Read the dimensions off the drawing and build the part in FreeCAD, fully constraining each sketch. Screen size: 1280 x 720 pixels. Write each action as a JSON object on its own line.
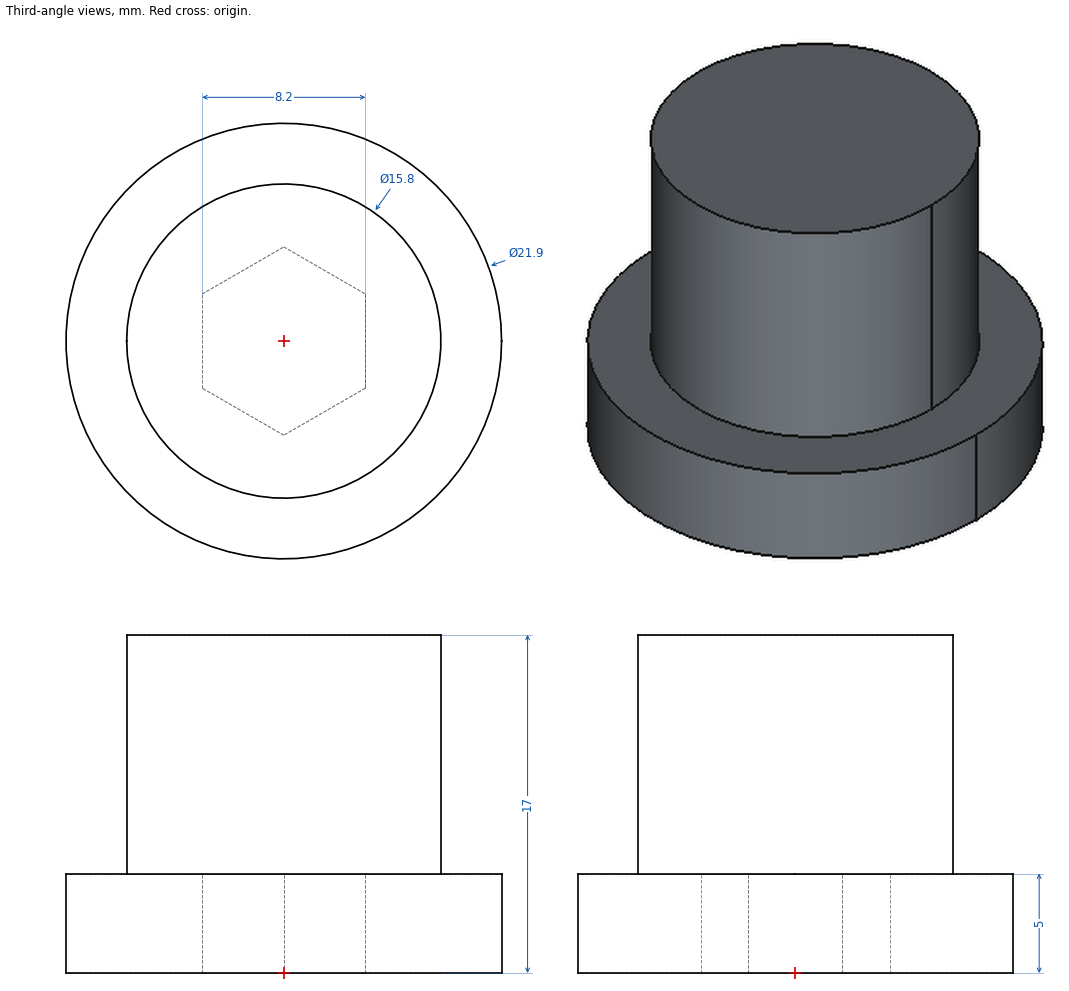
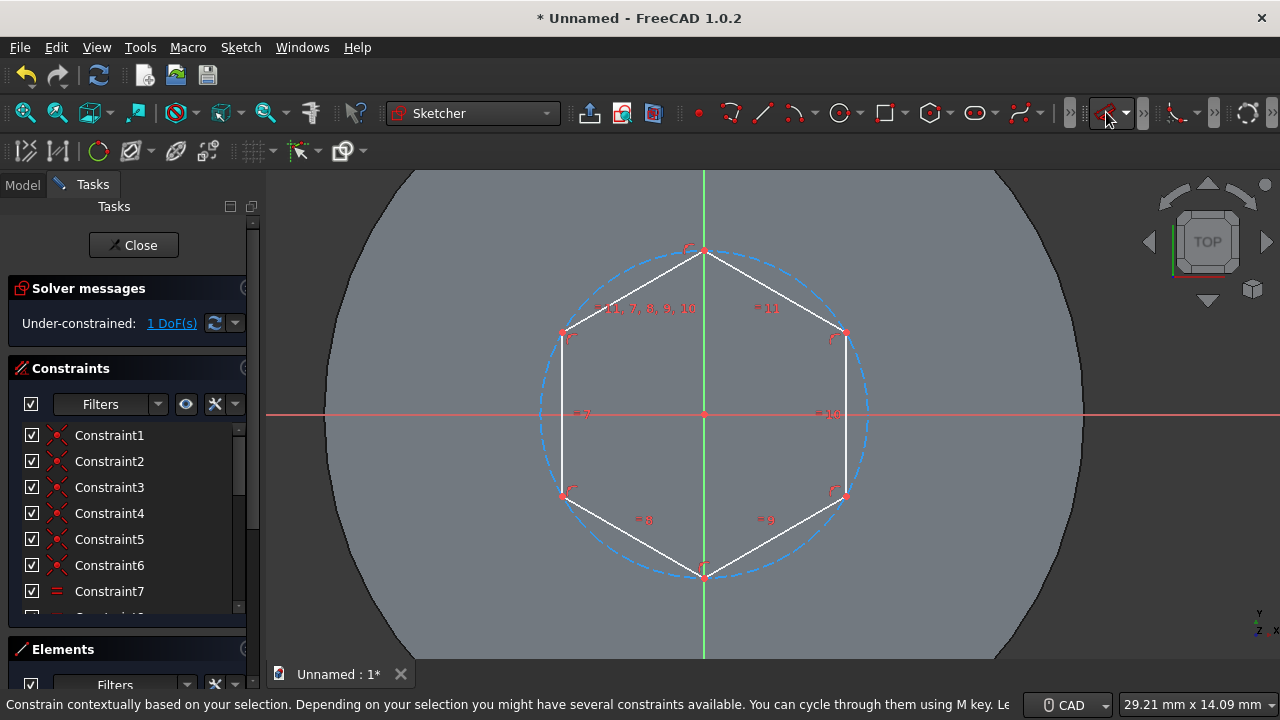
{"action": "left_click", "coordinate": [562, 333]}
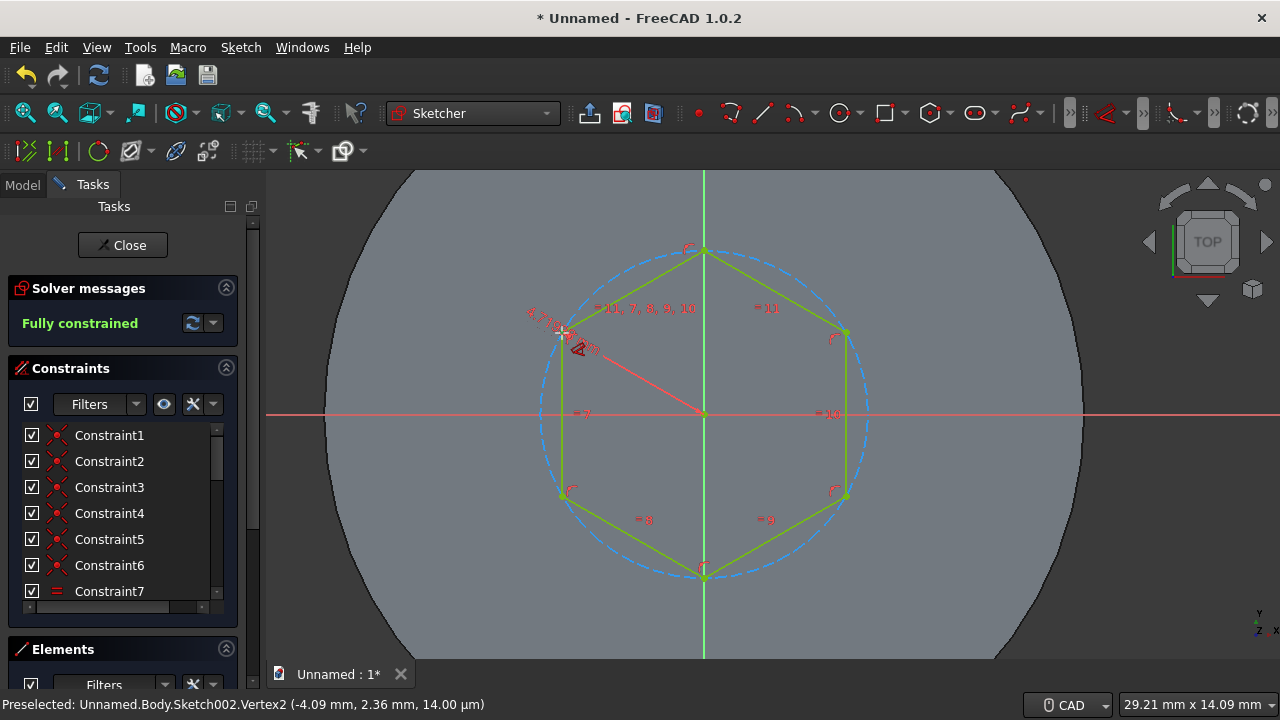
{"action": "left_click", "coordinate": [846, 496]}
{"action": "left_click", "coordinate": [605, 578]}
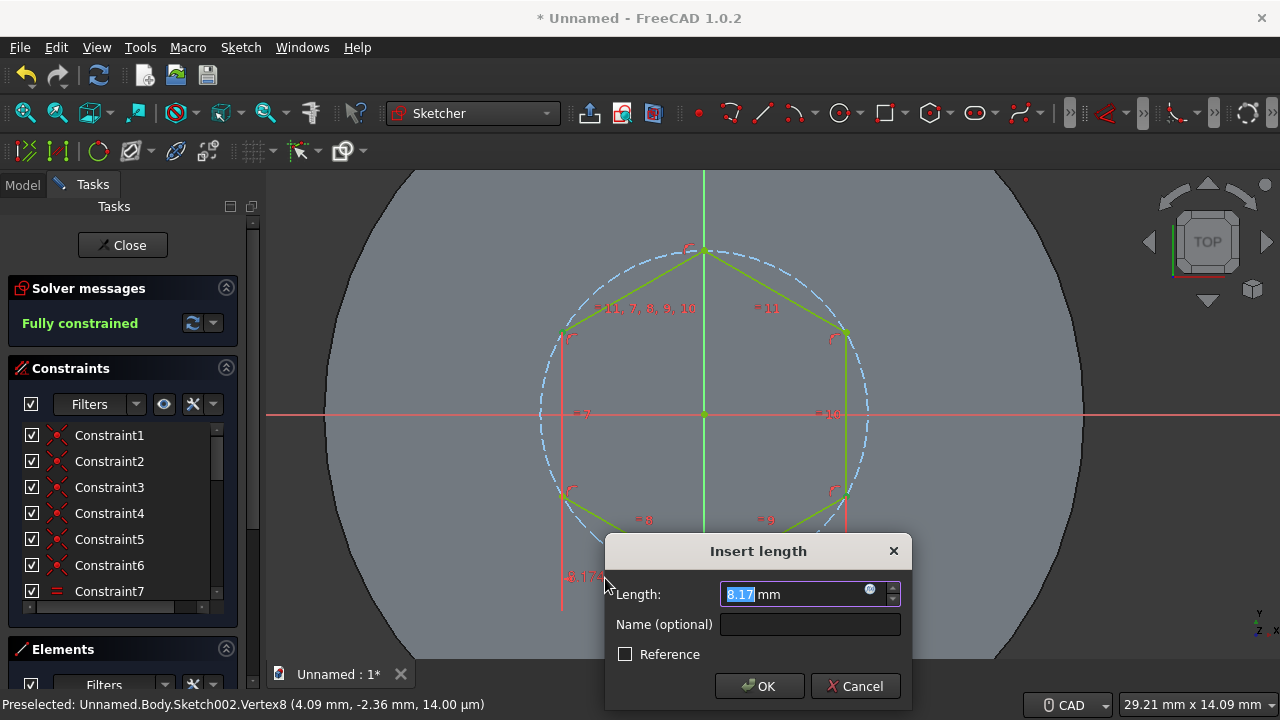
{"action": "type", "text": "8.2"}
{"action": "key", "text": "Return"}
{"action": "key", "text": "Escape"}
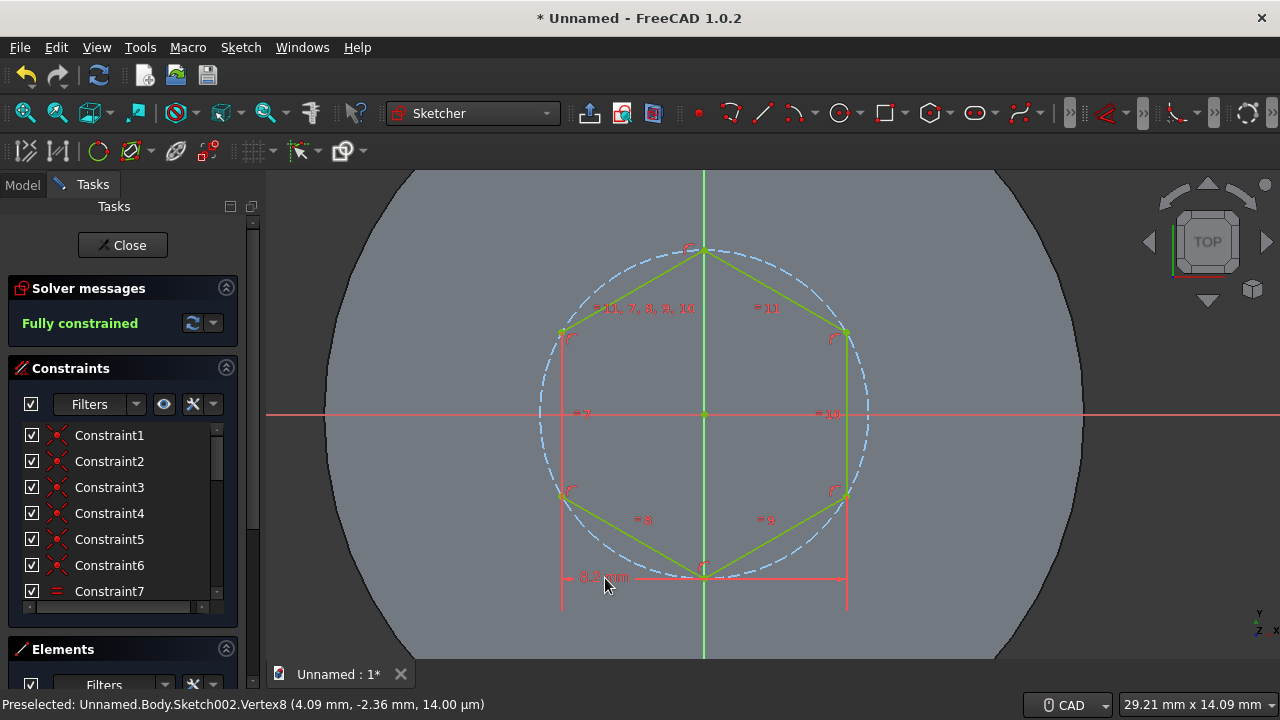
{"action": "left_click", "coordinate": [123, 245]}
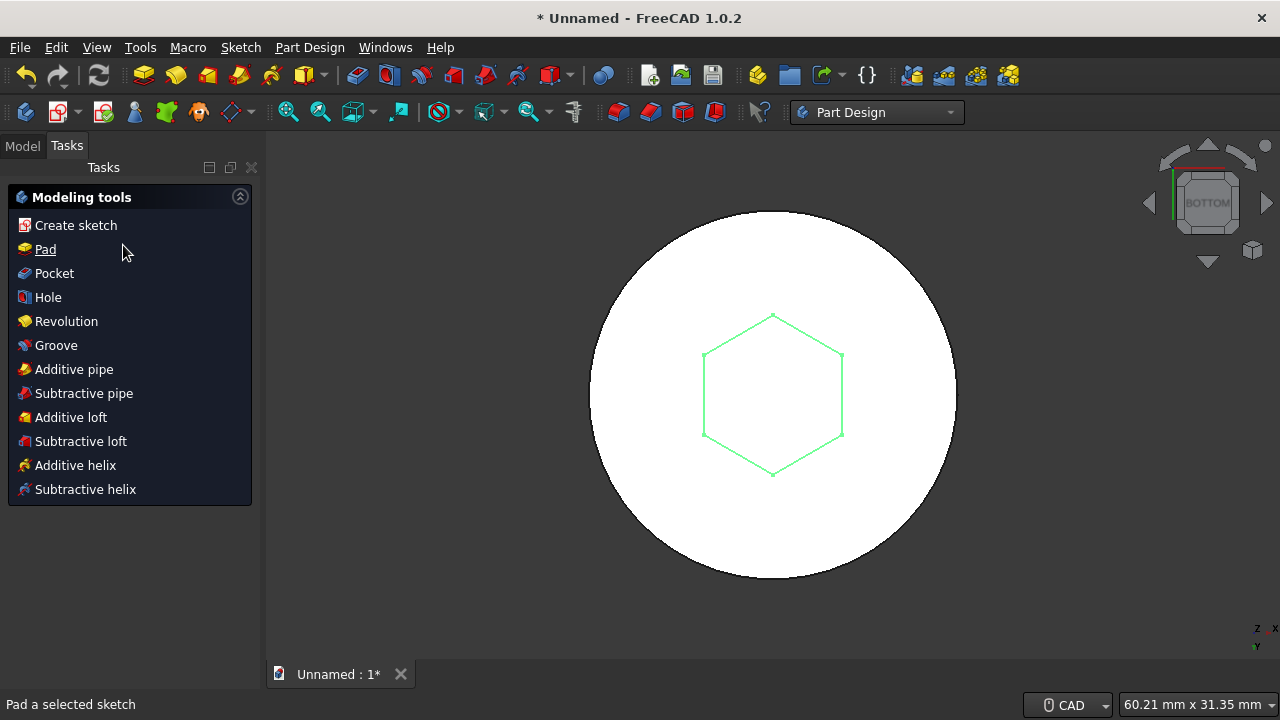
{"action": "left_click", "coordinate": [358, 76]}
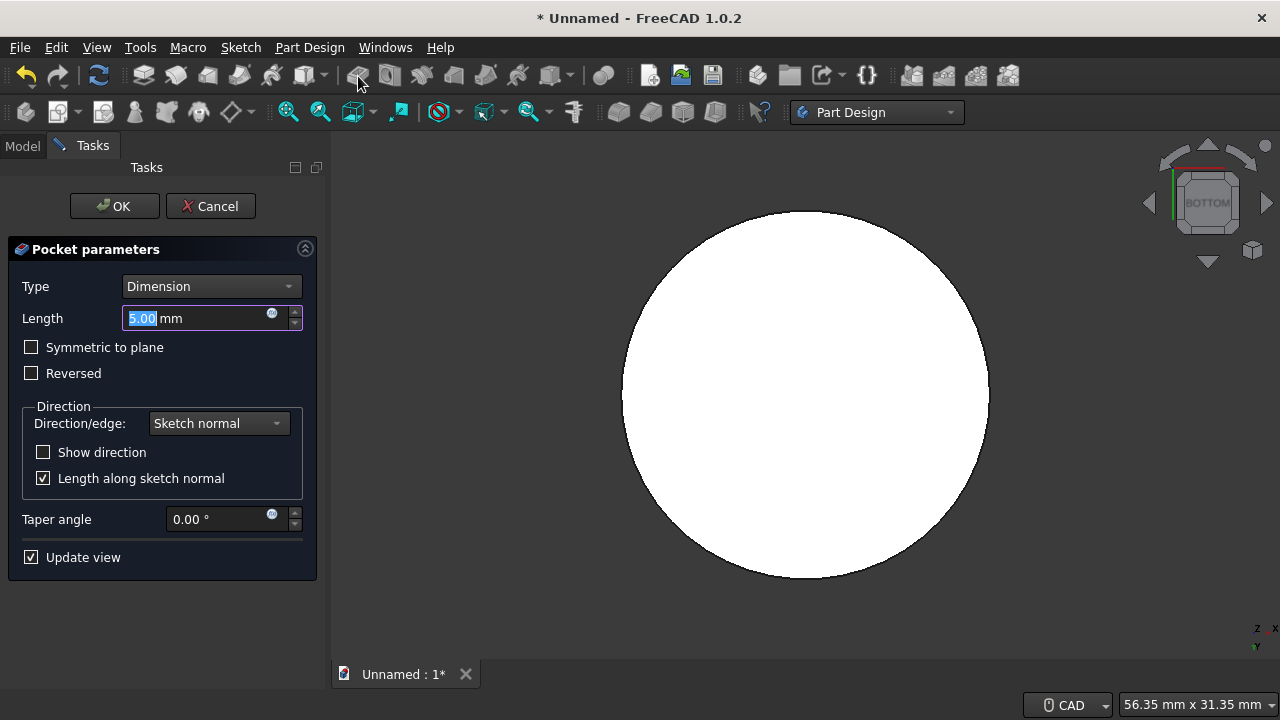
{"action": "type", "text": "5"}
{"action": "key", "text": "Tab"}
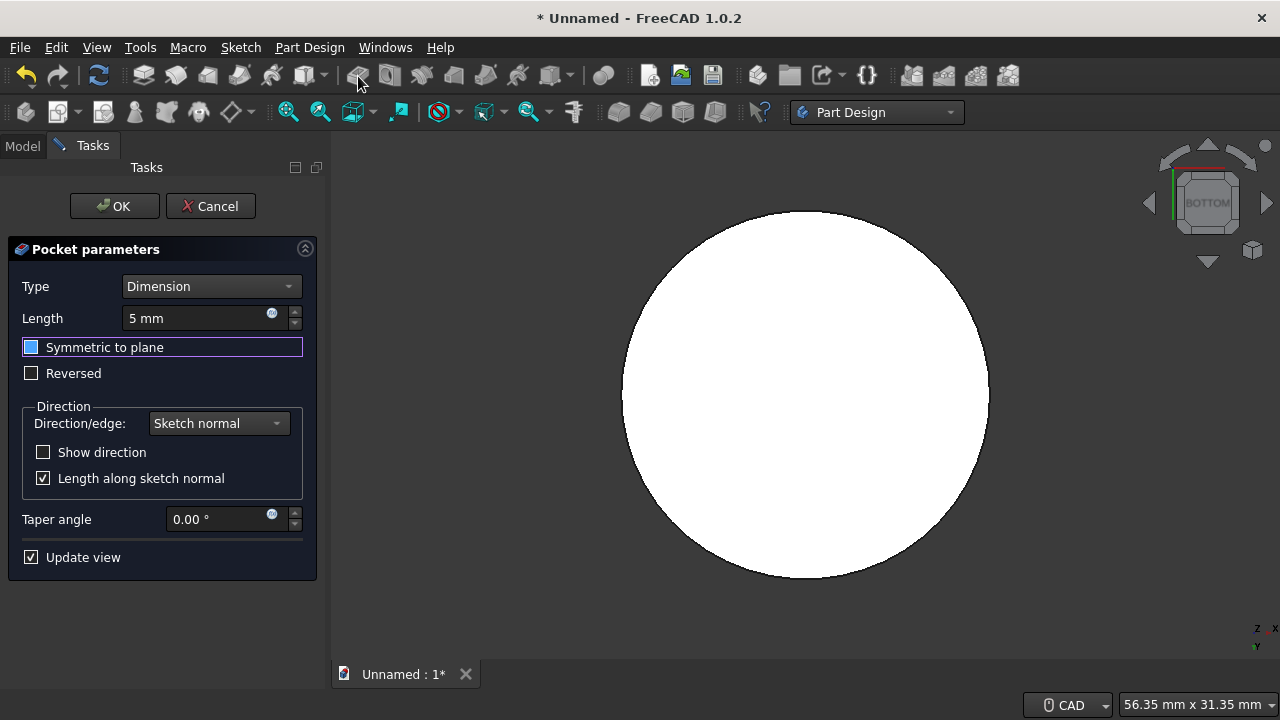
{"action": "left_click", "coordinate": [30, 373]}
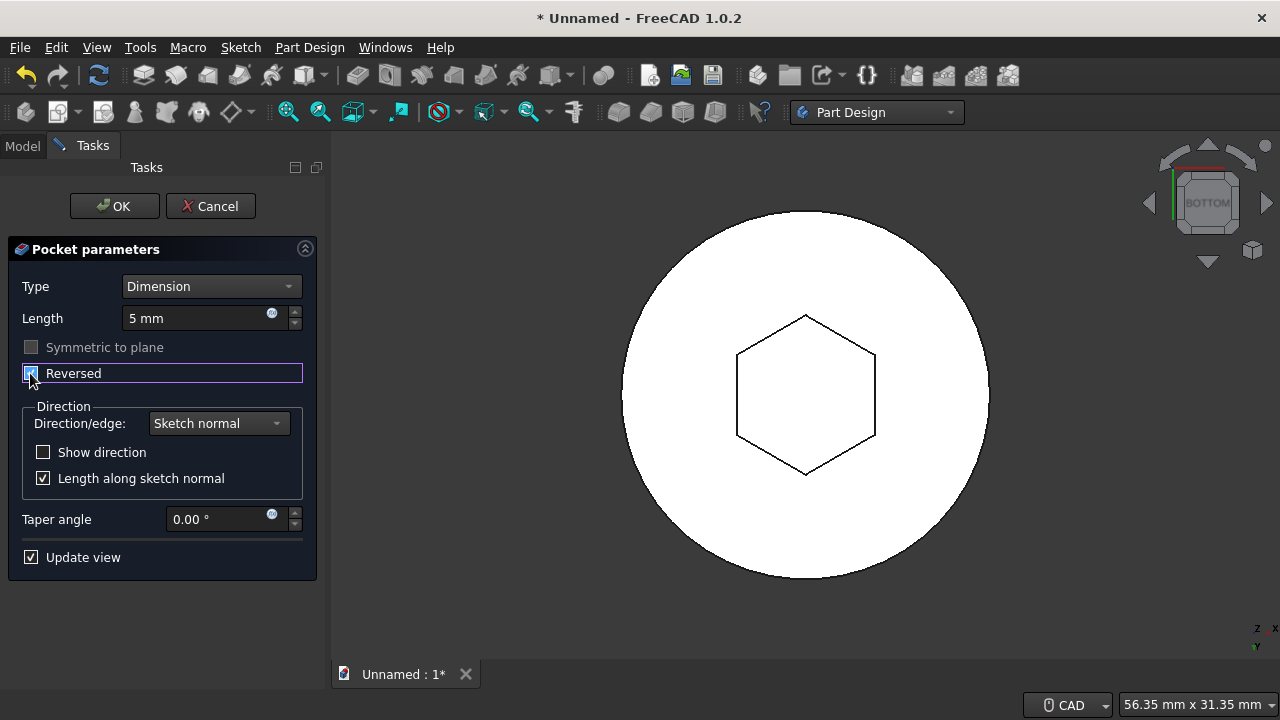
{"action": "left_click", "coordinate": [115, 206]}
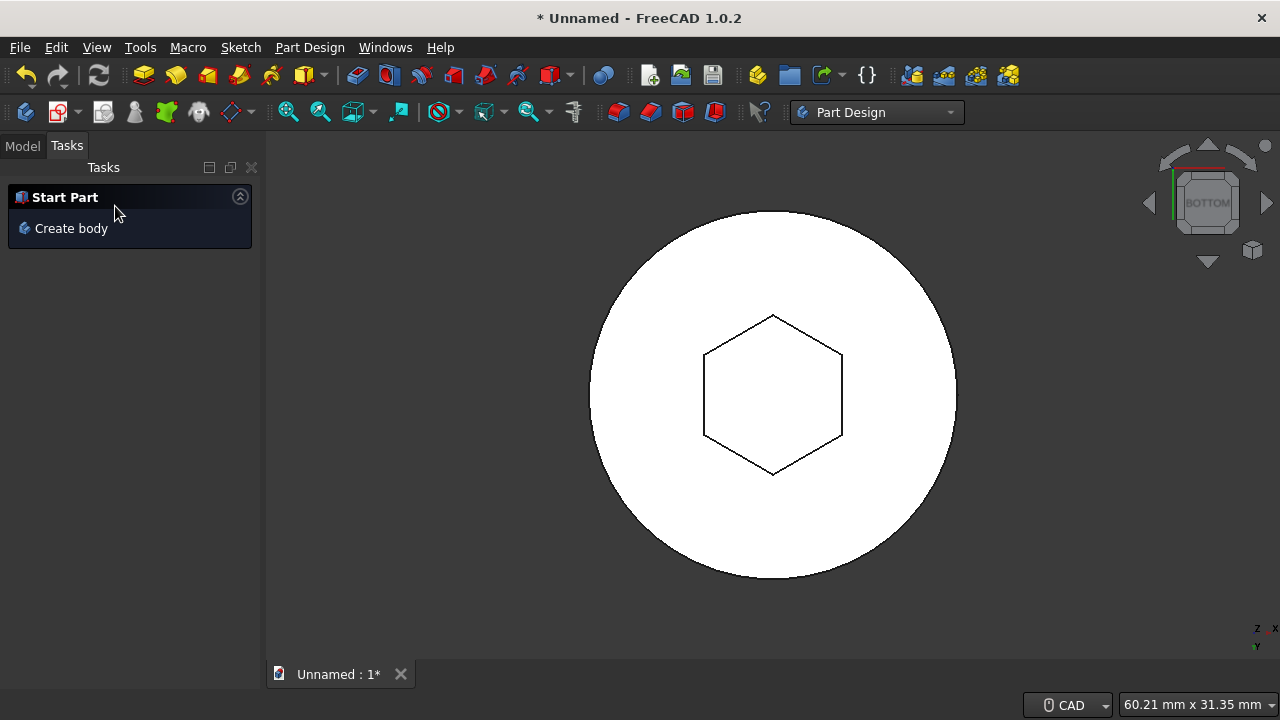
{"action": "key", "text": "0"}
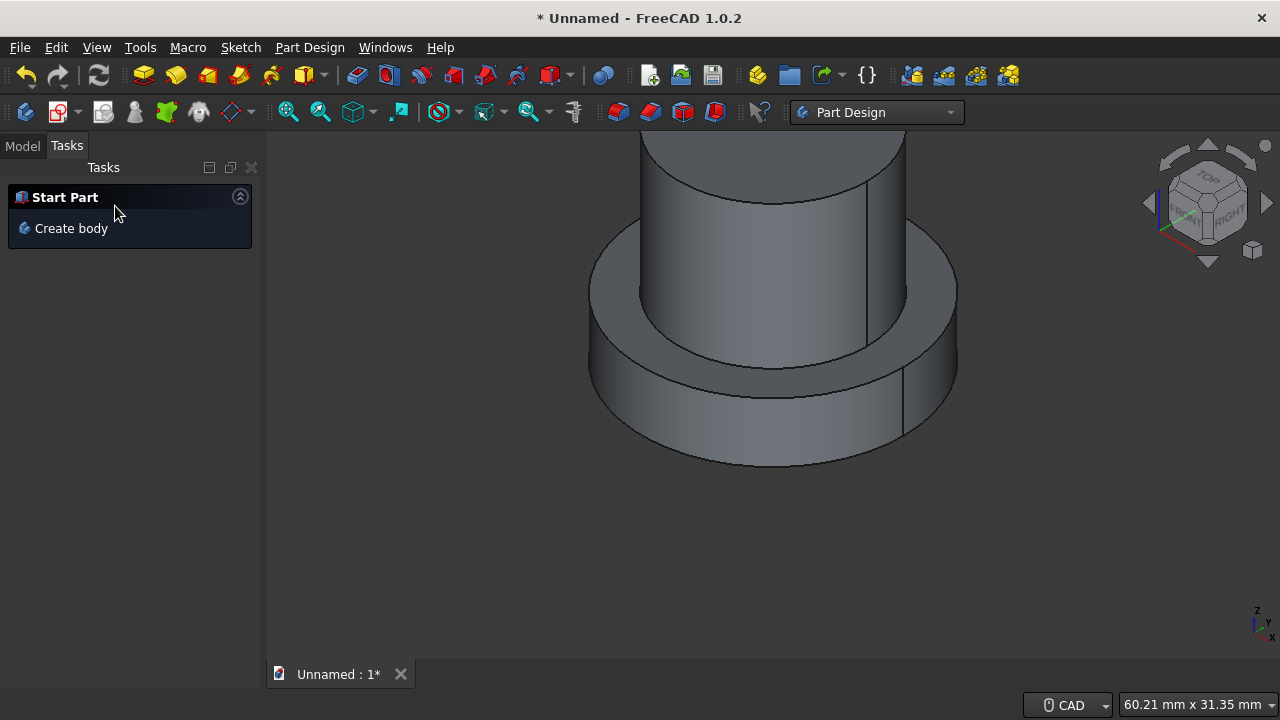
{"action": "left_click", "coordinate": [290, 112]}